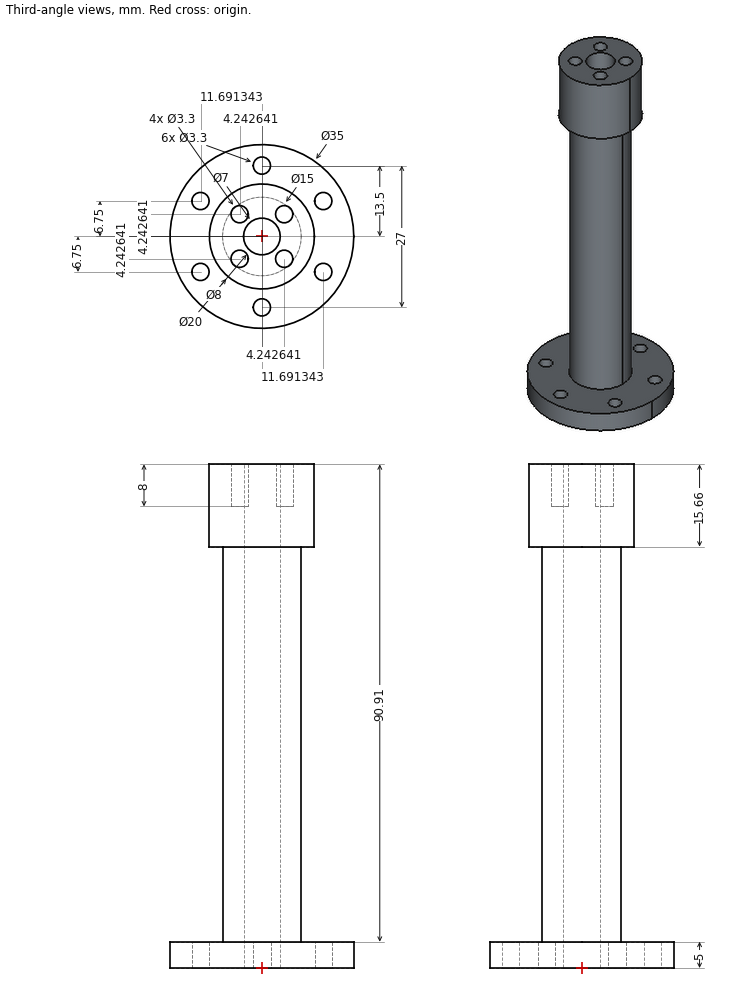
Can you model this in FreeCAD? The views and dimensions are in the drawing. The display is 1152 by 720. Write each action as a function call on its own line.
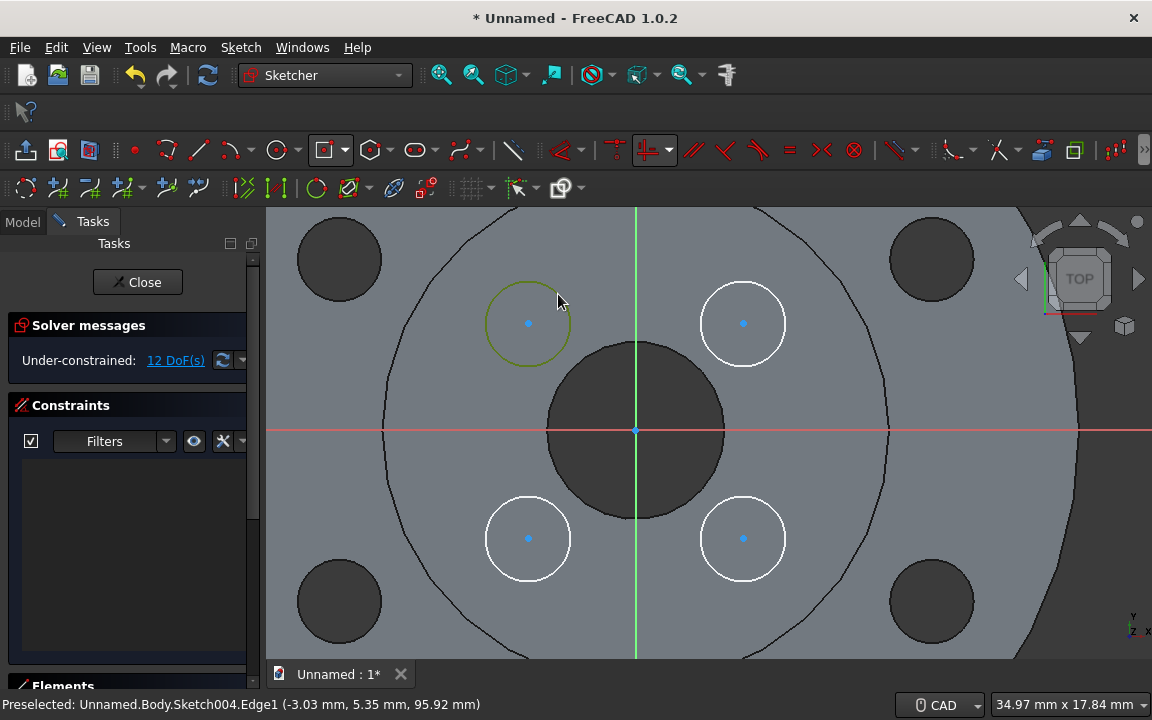
click(558, 509)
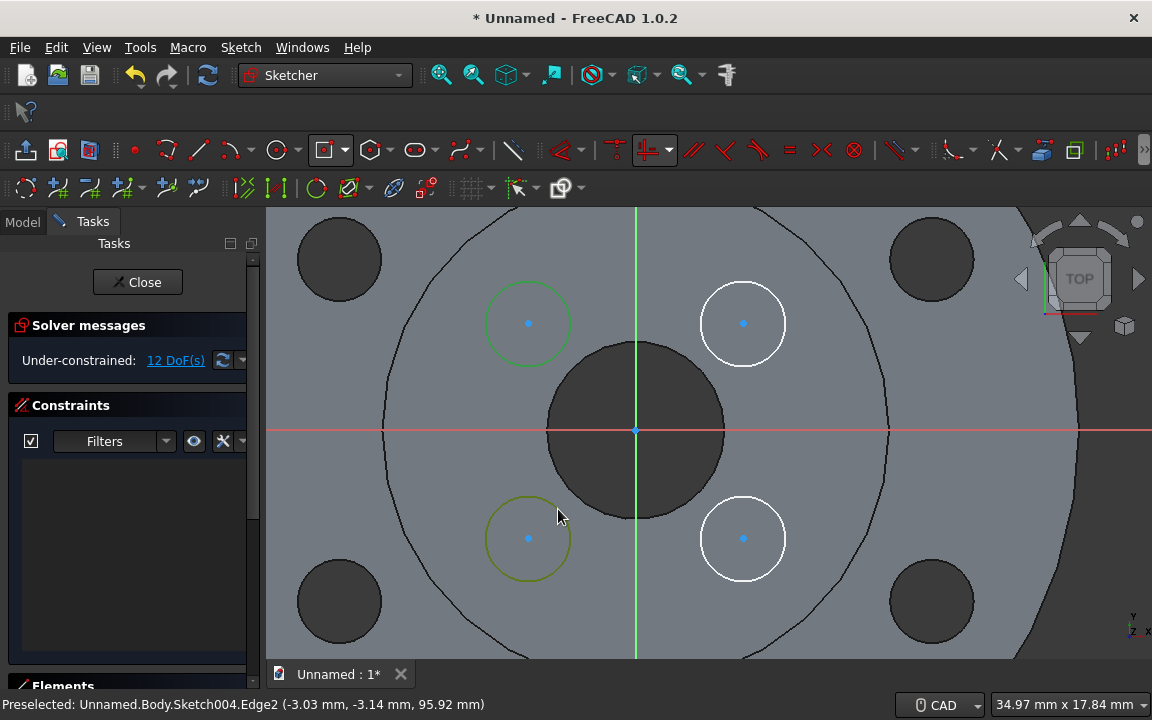
click(773, 509)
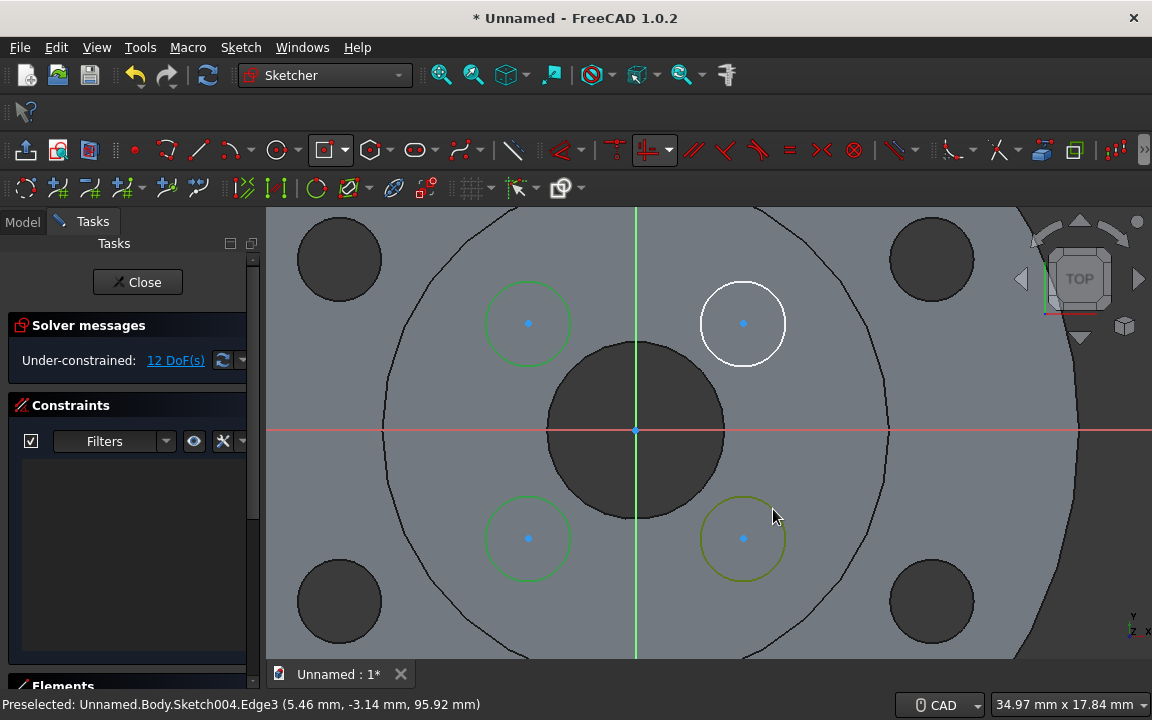
click(773, 294)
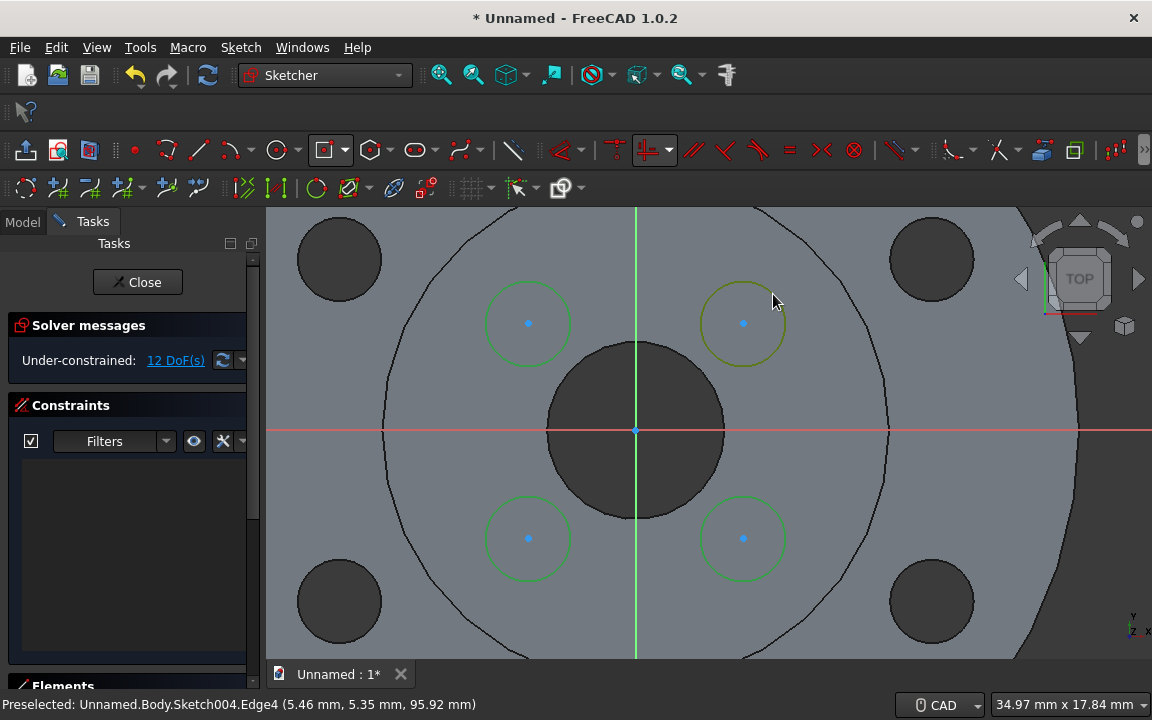
click(790, 150)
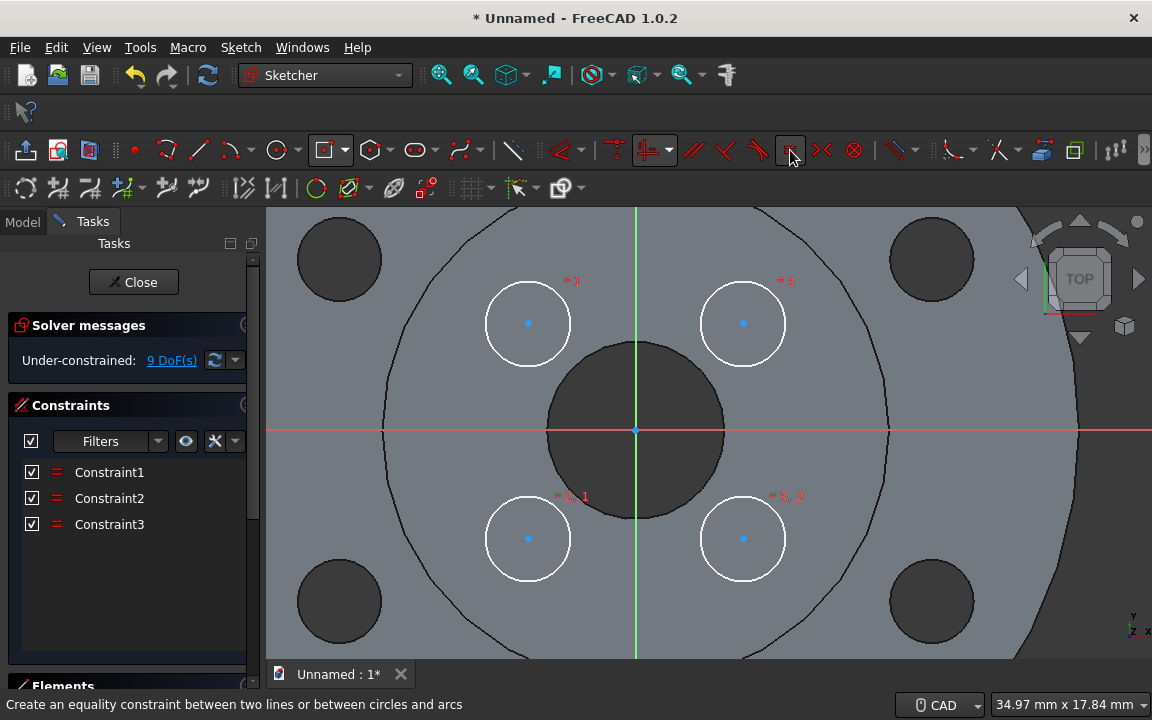
click(528, 324)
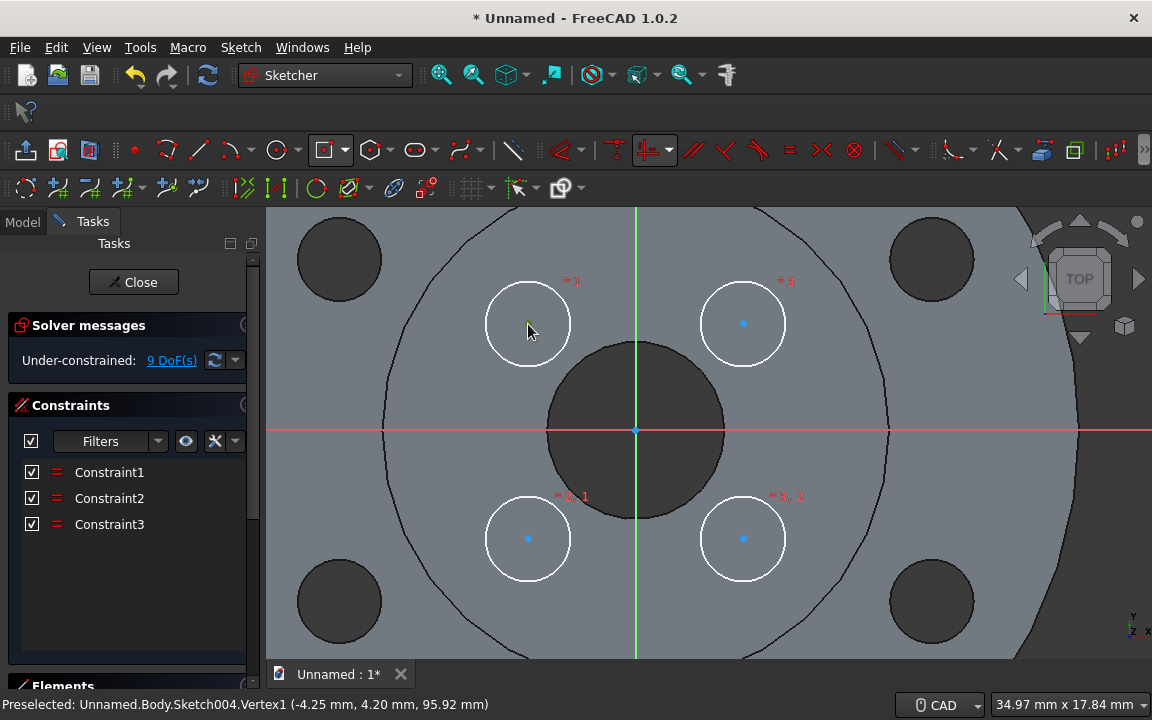
click(528, 539)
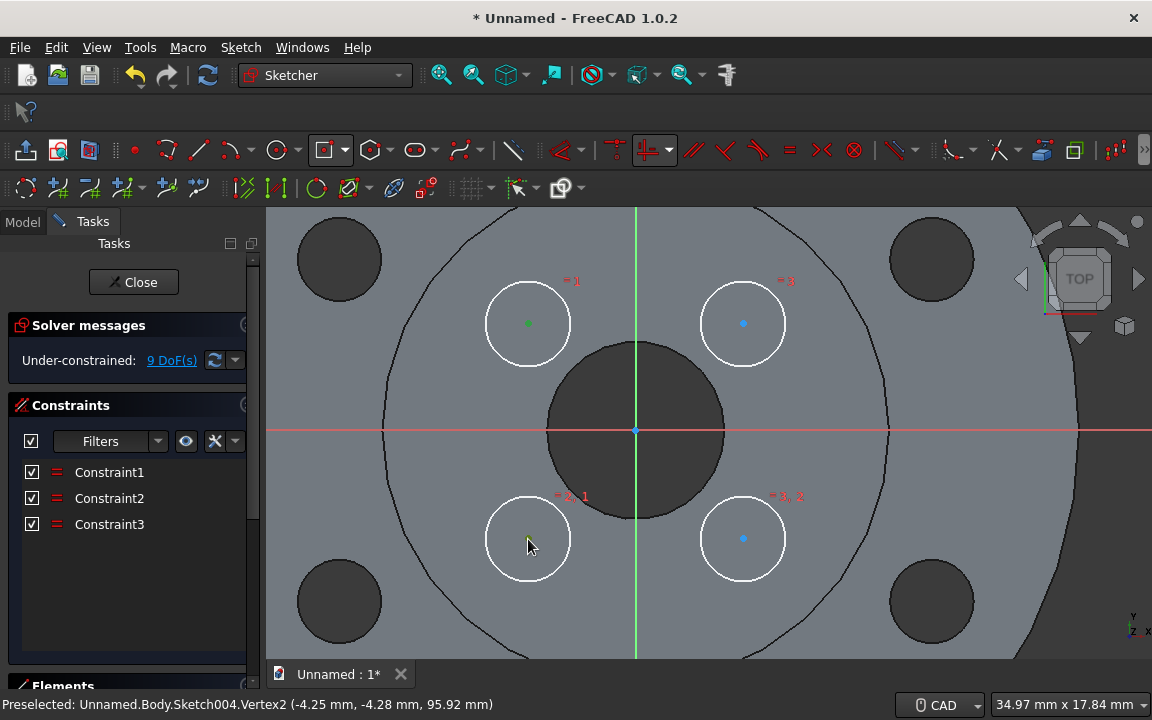
key(v)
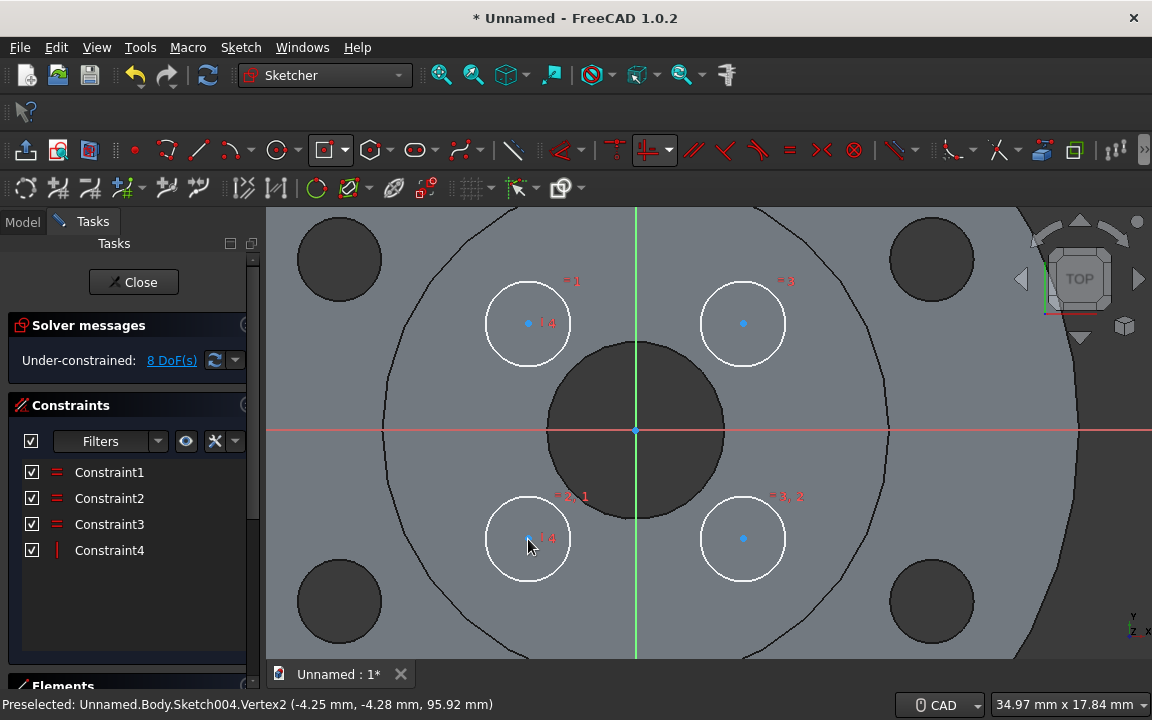
click(528, 539)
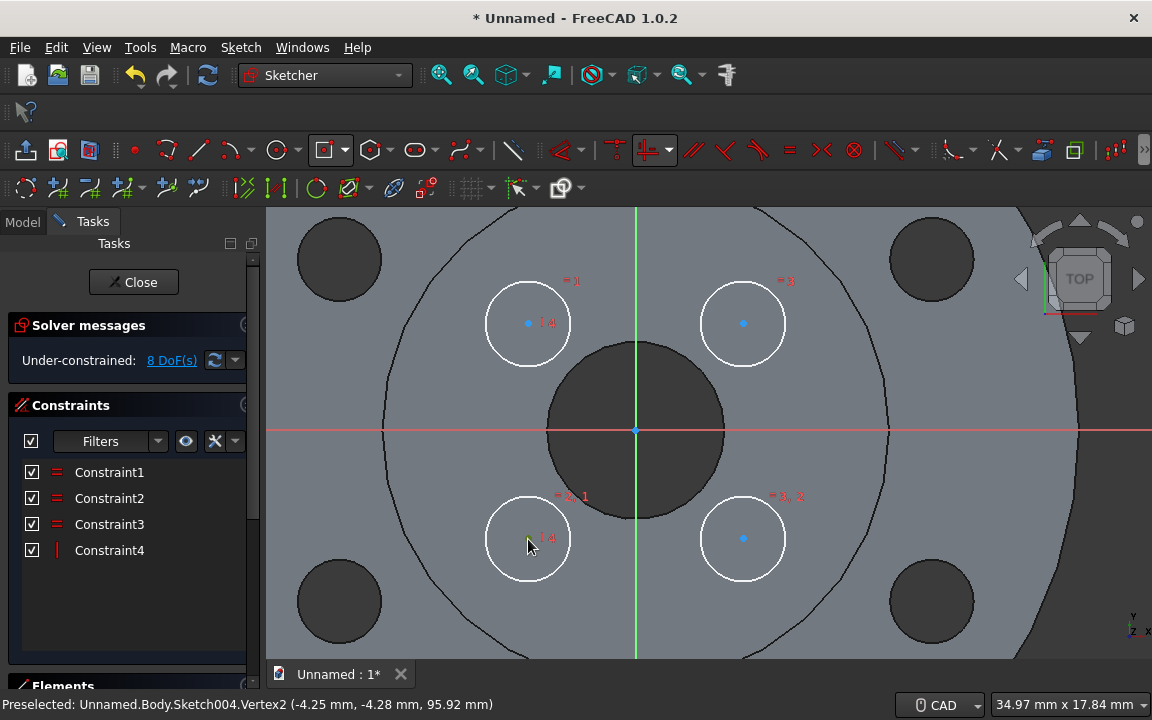
click(743, 539)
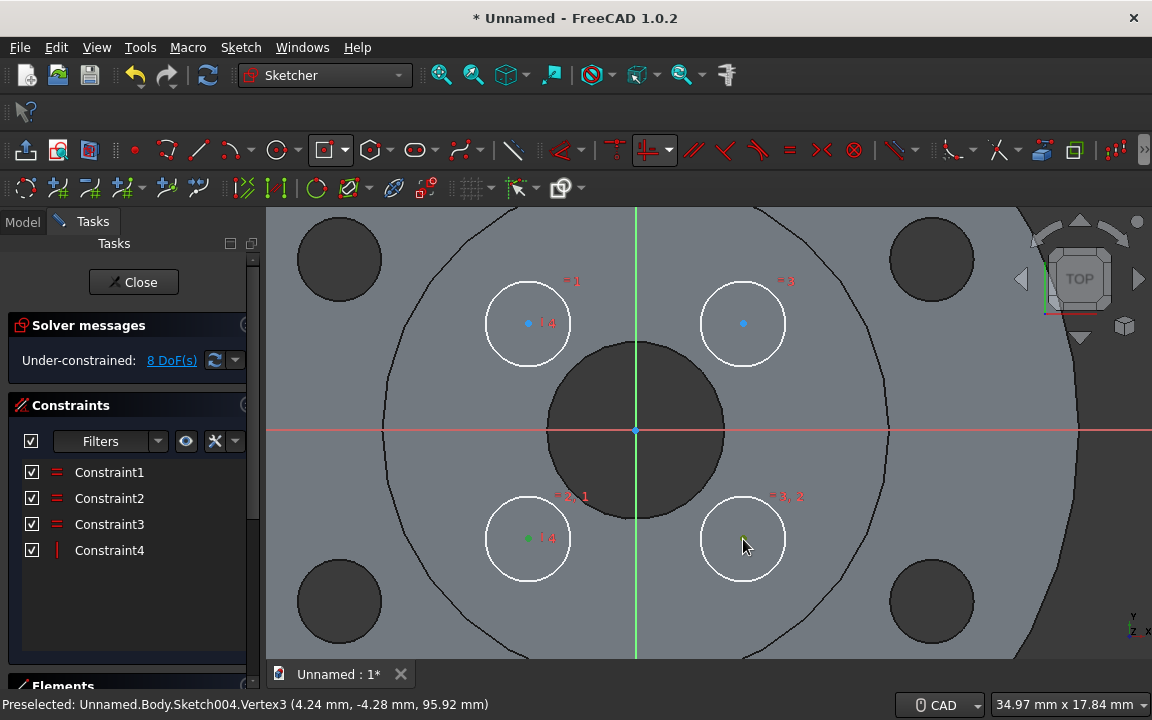
key(h)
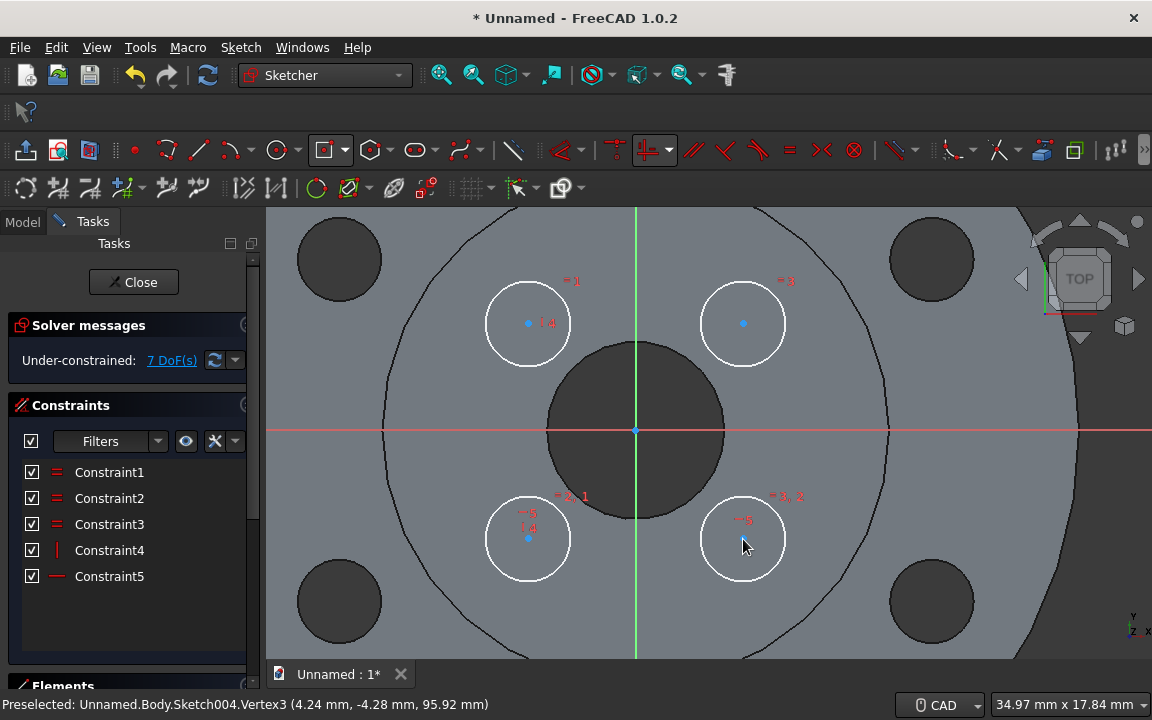
click(743, 539)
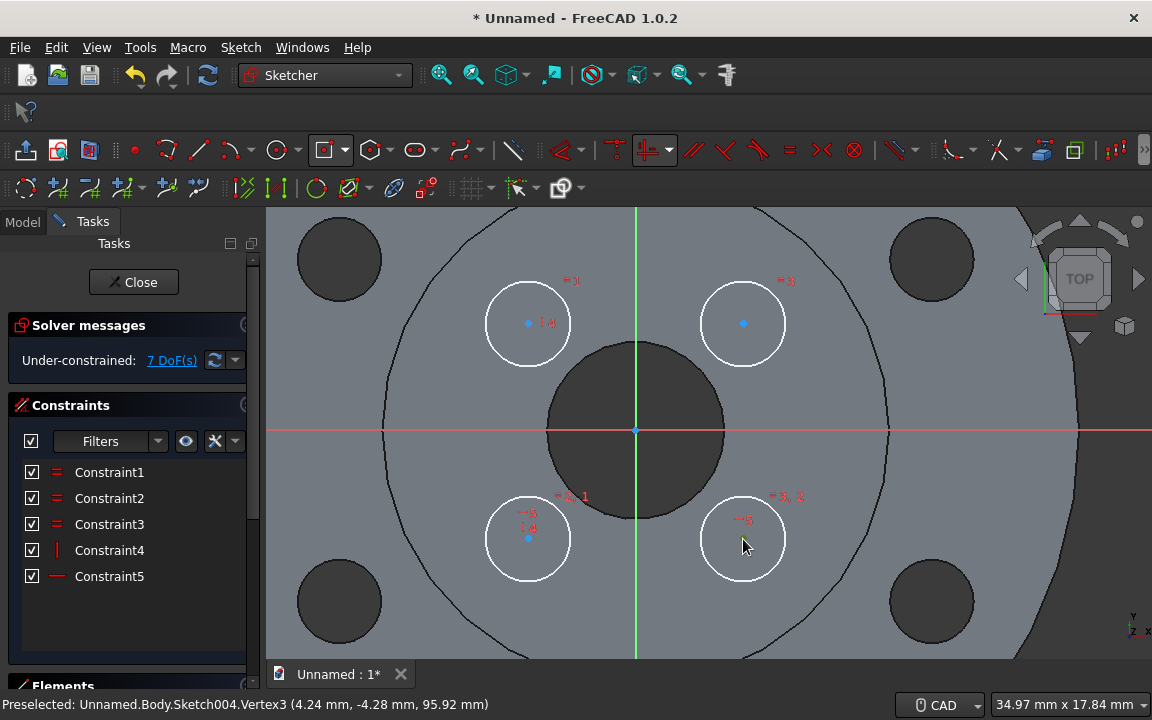
click(743, 324)